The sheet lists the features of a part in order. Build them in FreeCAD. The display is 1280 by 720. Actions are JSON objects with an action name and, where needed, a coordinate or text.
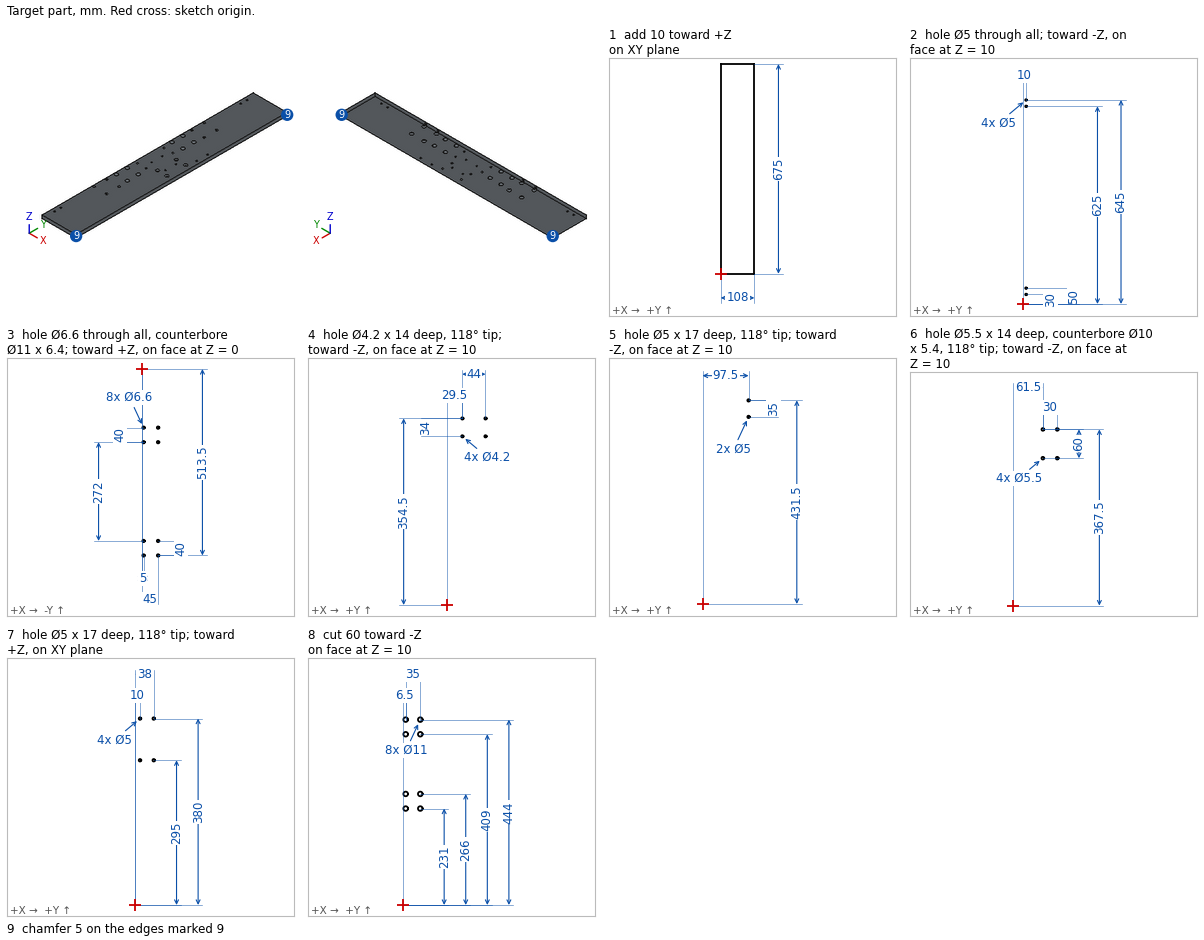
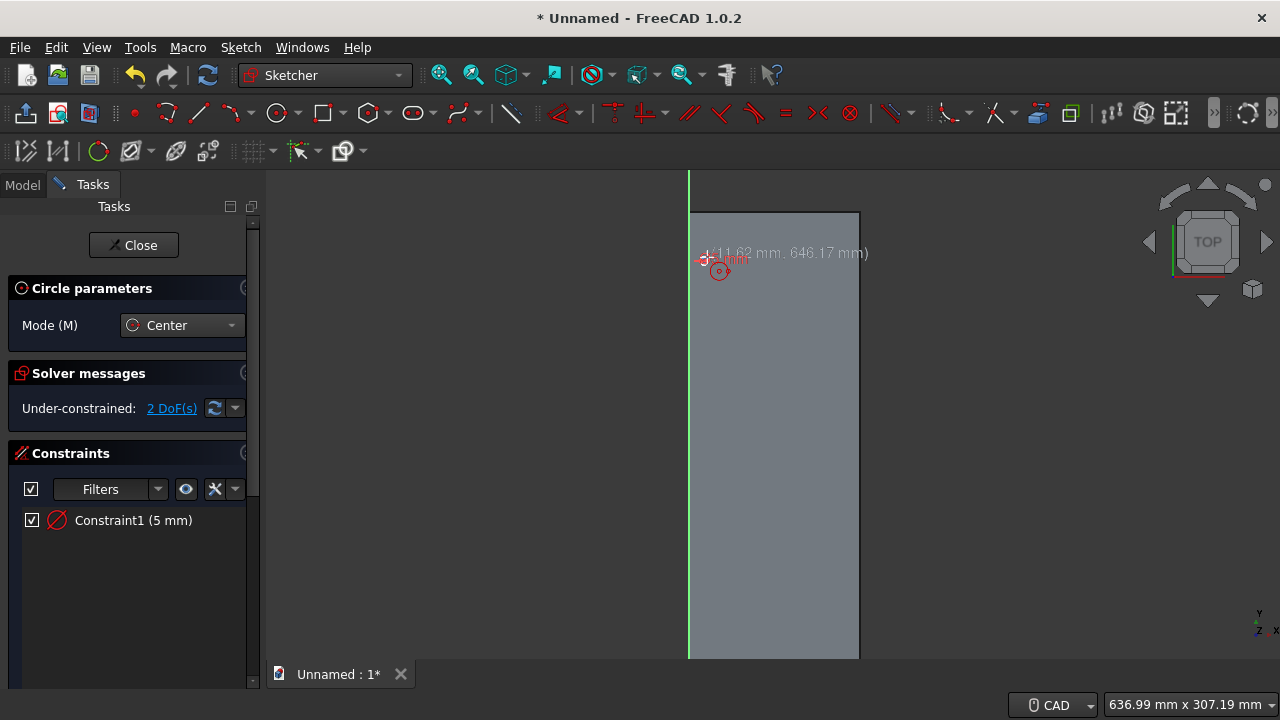
{"action": "scroll", "coordinate": [704, 292], "scroll_direction": "up", "scroll_amount": 9}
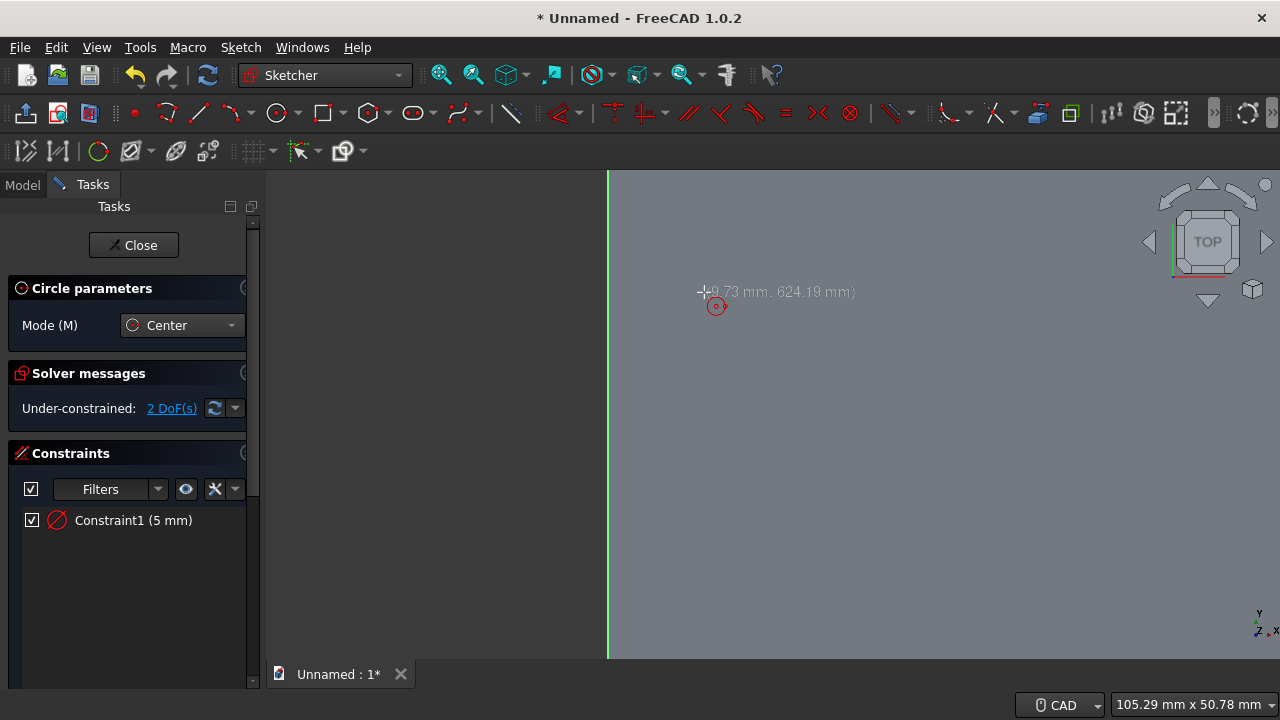
{"action": "scroll", "coordinate": [706, 269], "scroll_direction": "down", "scroll_amount": 15}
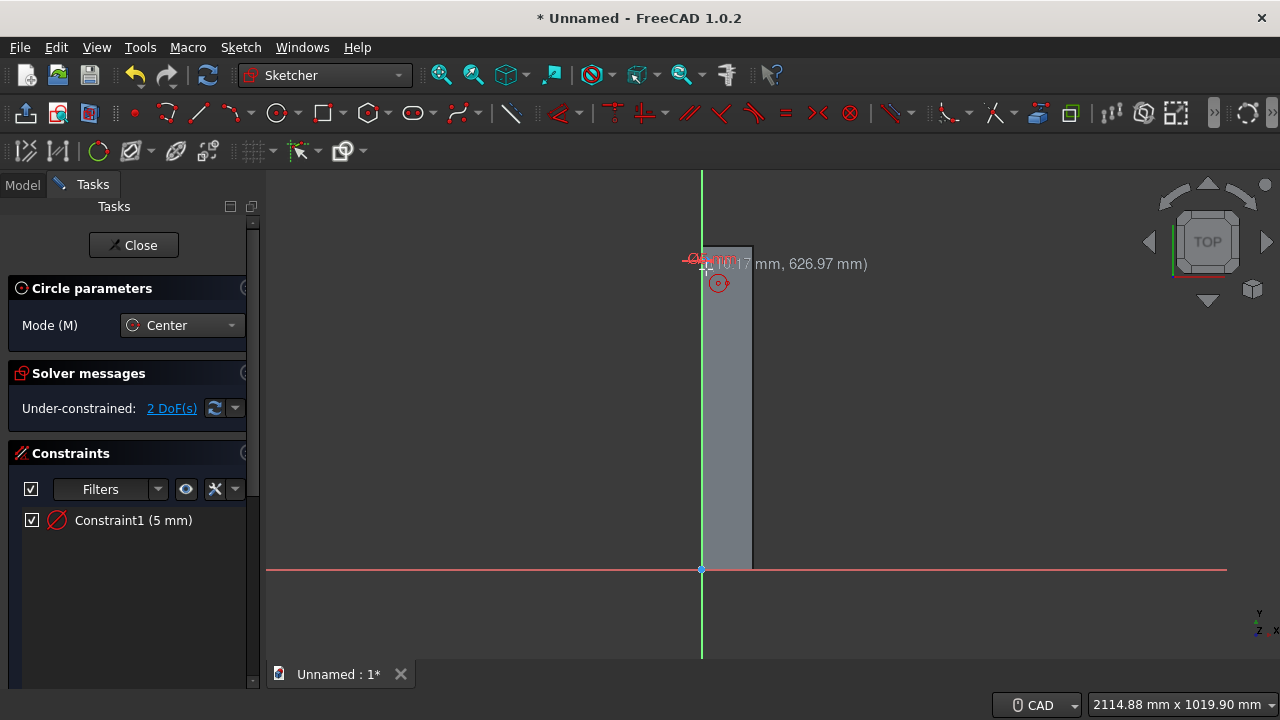
{"action": "scroll", "coordinate": [706, 270], "scroll_direction": "up", "scroll_amount": 6}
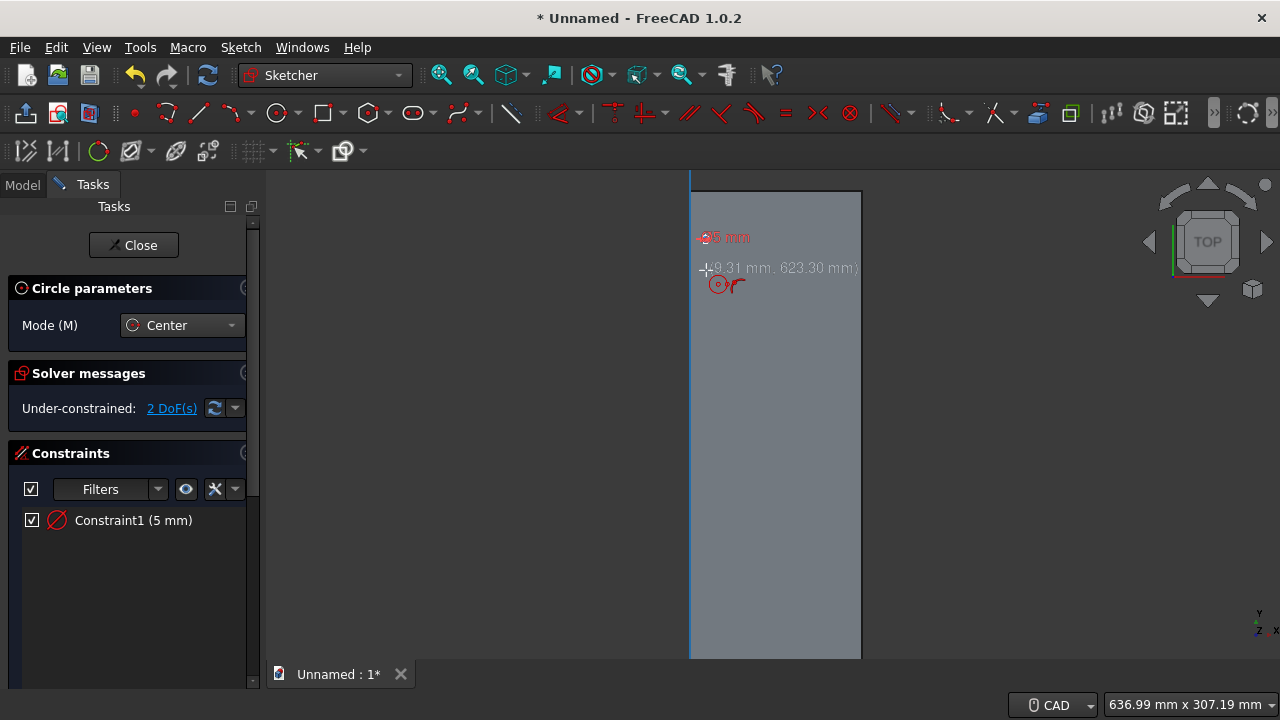
{"action": "left_click", "coordinate": [706, 270]}
{"action": "mouse_move", "coordinate": [709, 267]}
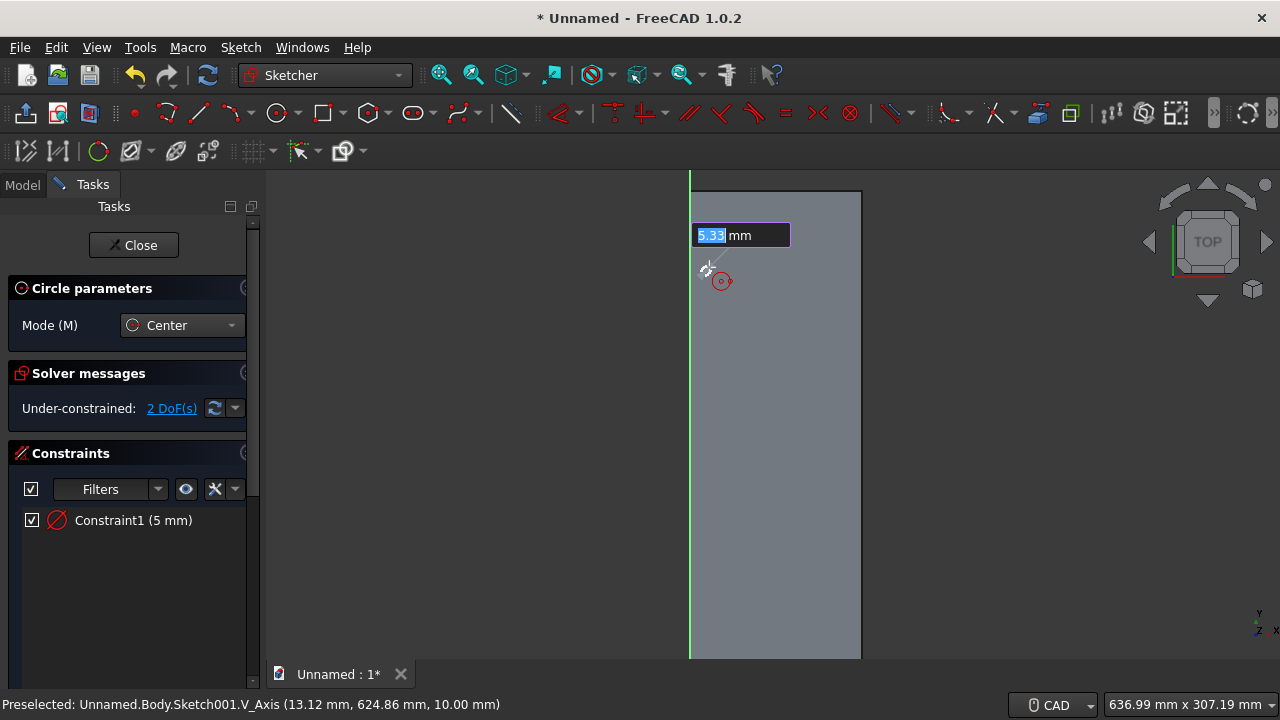
{"action": "type", "text": "5"}
{"action": "key", "text": "Return"}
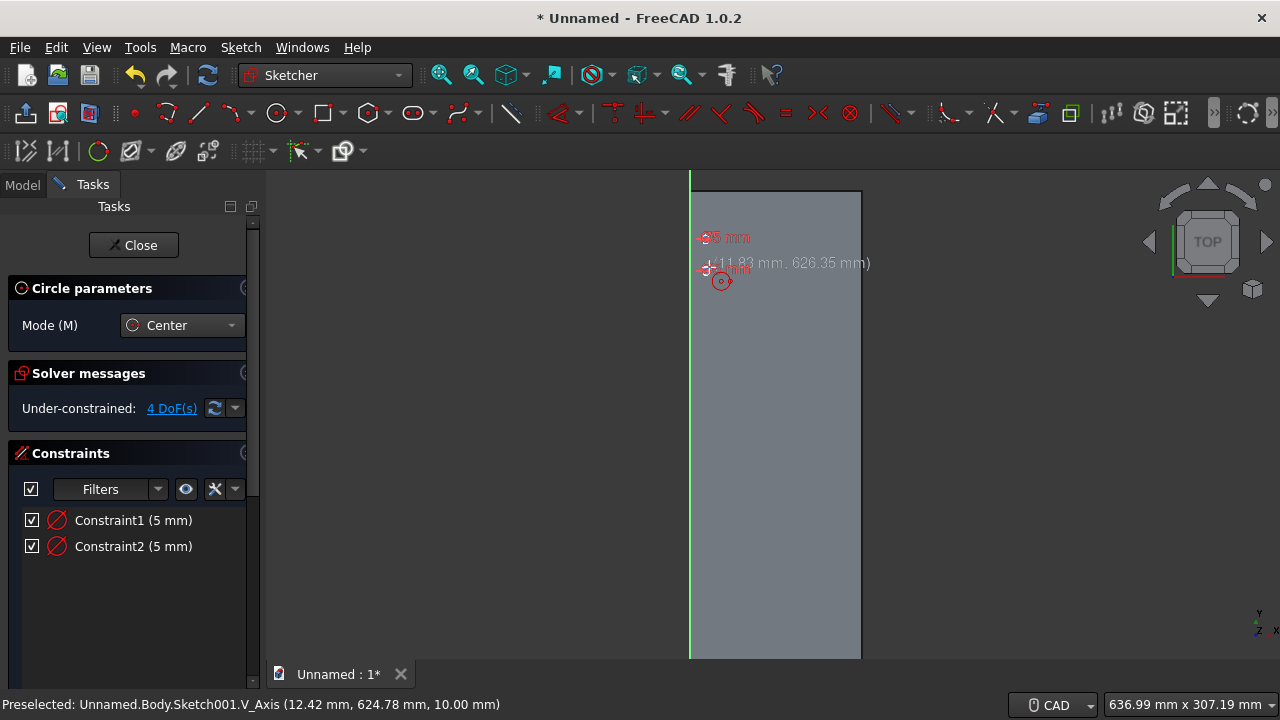
{"action": "scroll", "coordinate": [706, 270], "scroll_direction": "down", "scroll_amount": 6}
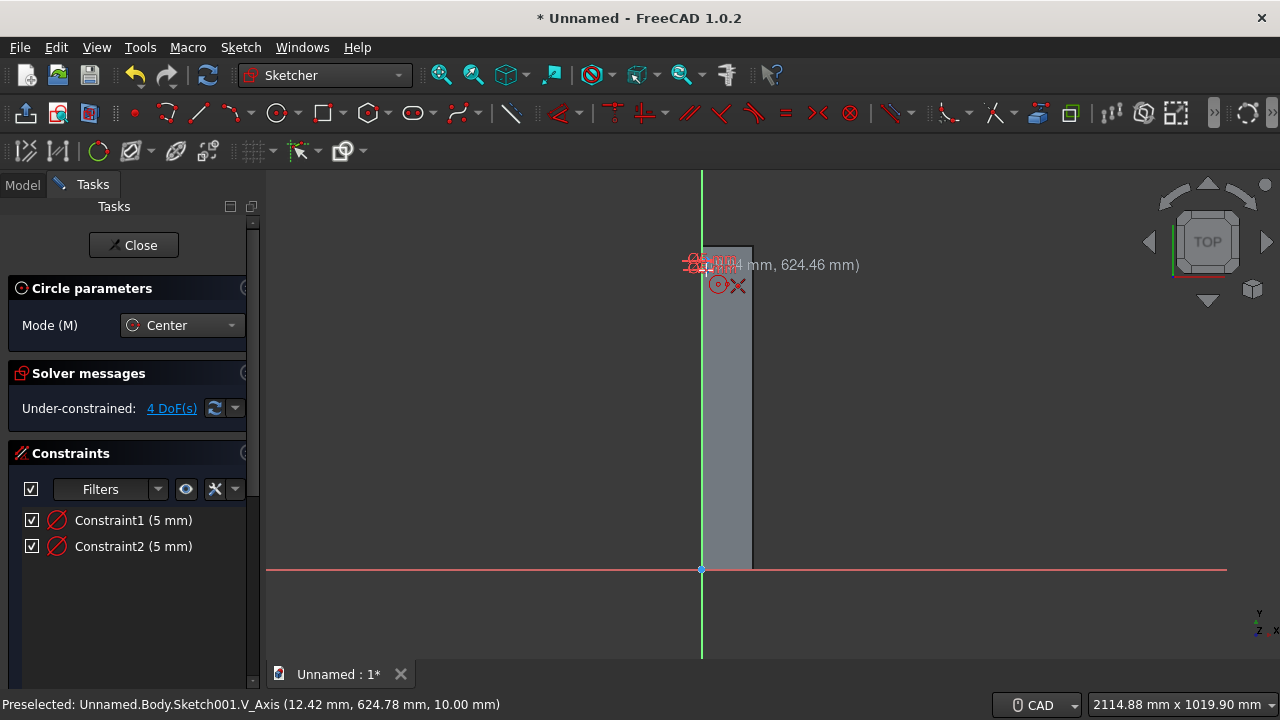
{"action": "scroll", "coordinate": [706, 546], "scroll_direction": "up", "scroll_amount": 15}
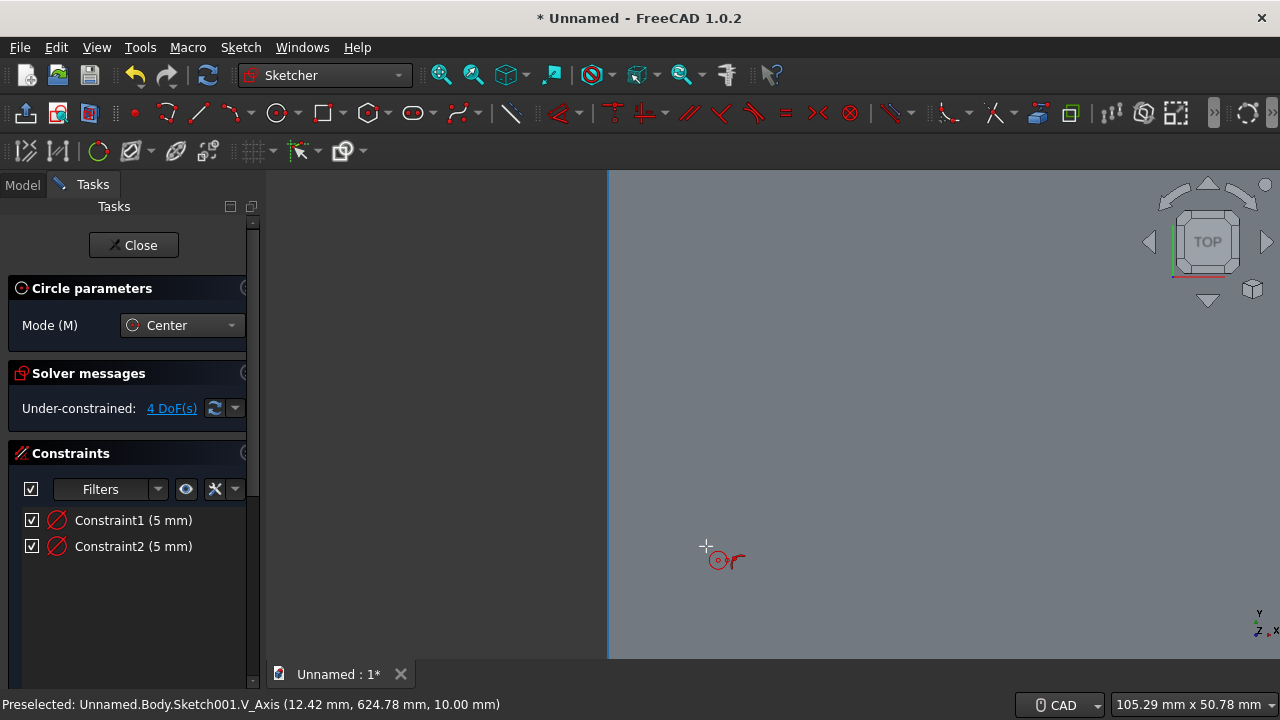
{"action": "scroll", "coordinate": [706, 547], "scroll_direction": "down", "scroll_amount": 15}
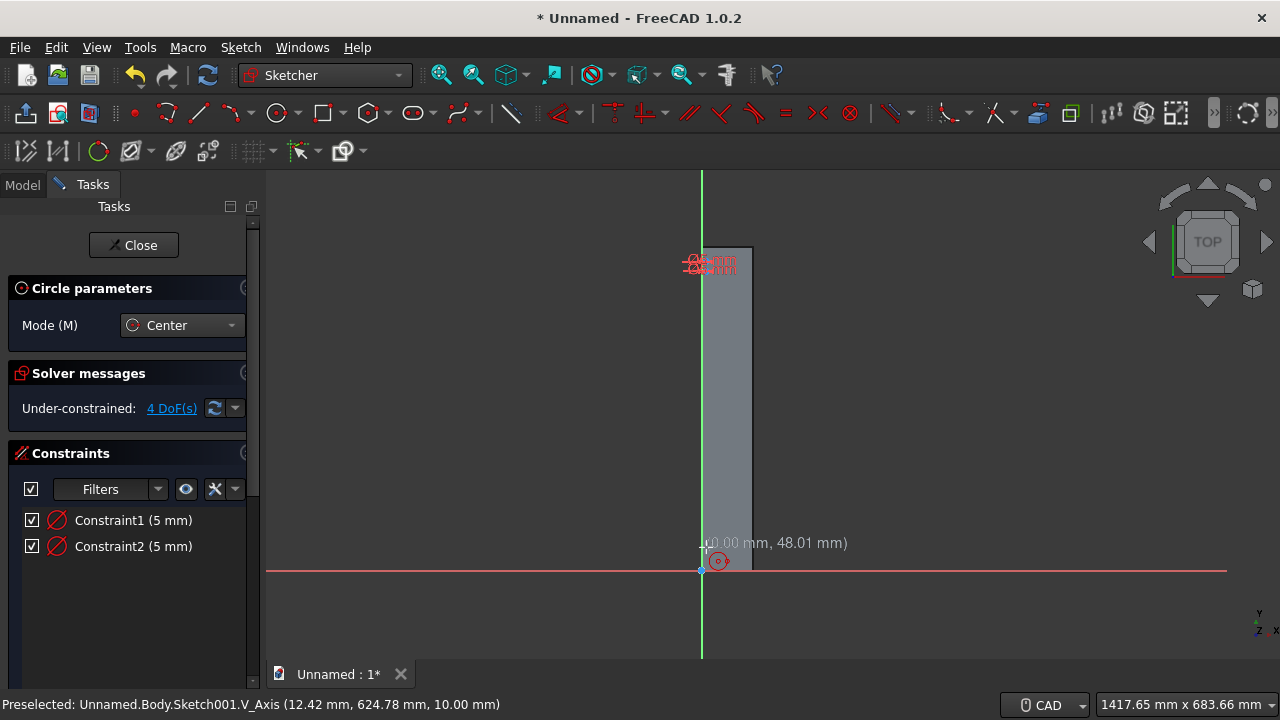
{"action": "scroll", "coordinate": [706, 547], "scroll_direction": "up", "scroll_amount": 6}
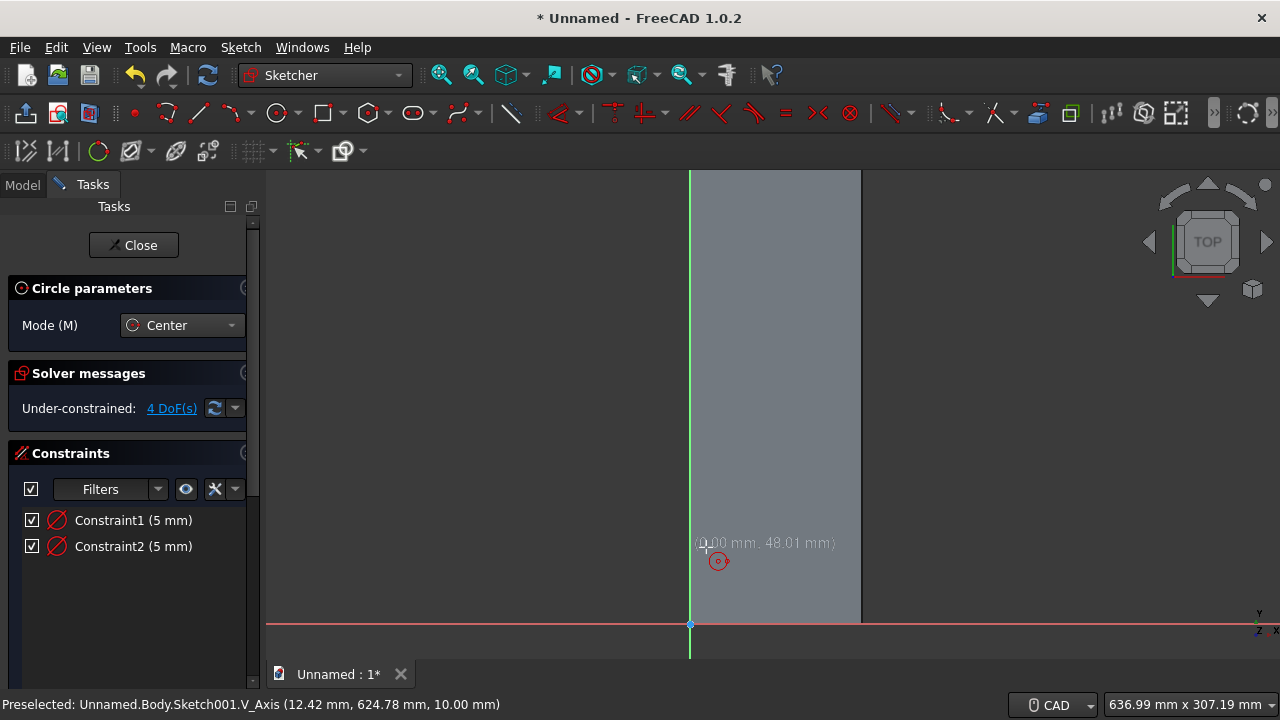
{"action": "left_click", "coordinate": [706, 545]}
{"action": "mouse_move", "coordinate": [709, 542]}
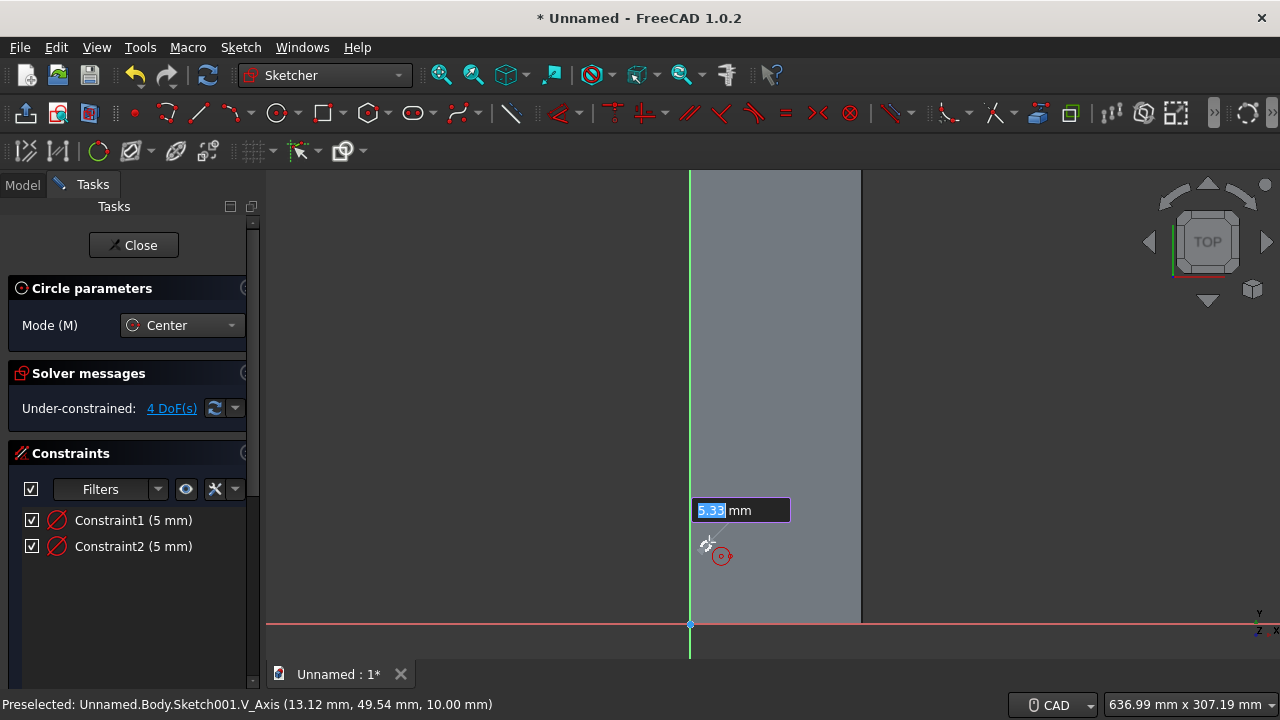
{"action": "type", "text": "5"}
{"action": "key", "text": "Return"}